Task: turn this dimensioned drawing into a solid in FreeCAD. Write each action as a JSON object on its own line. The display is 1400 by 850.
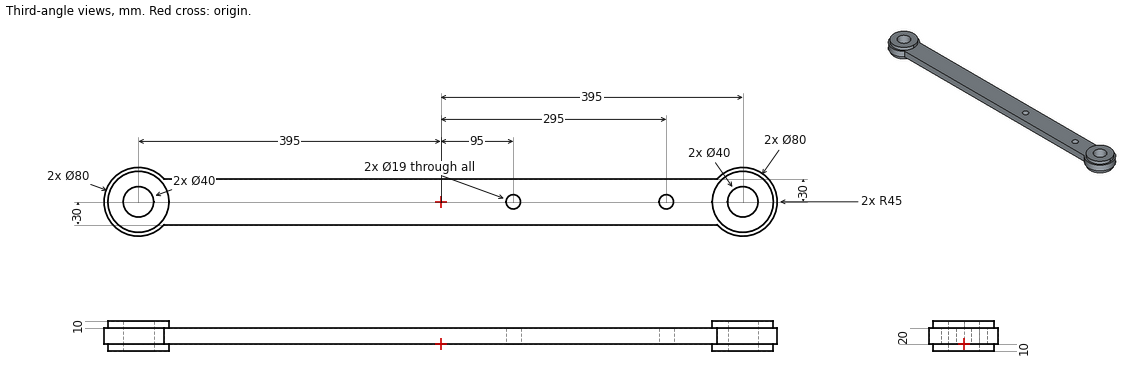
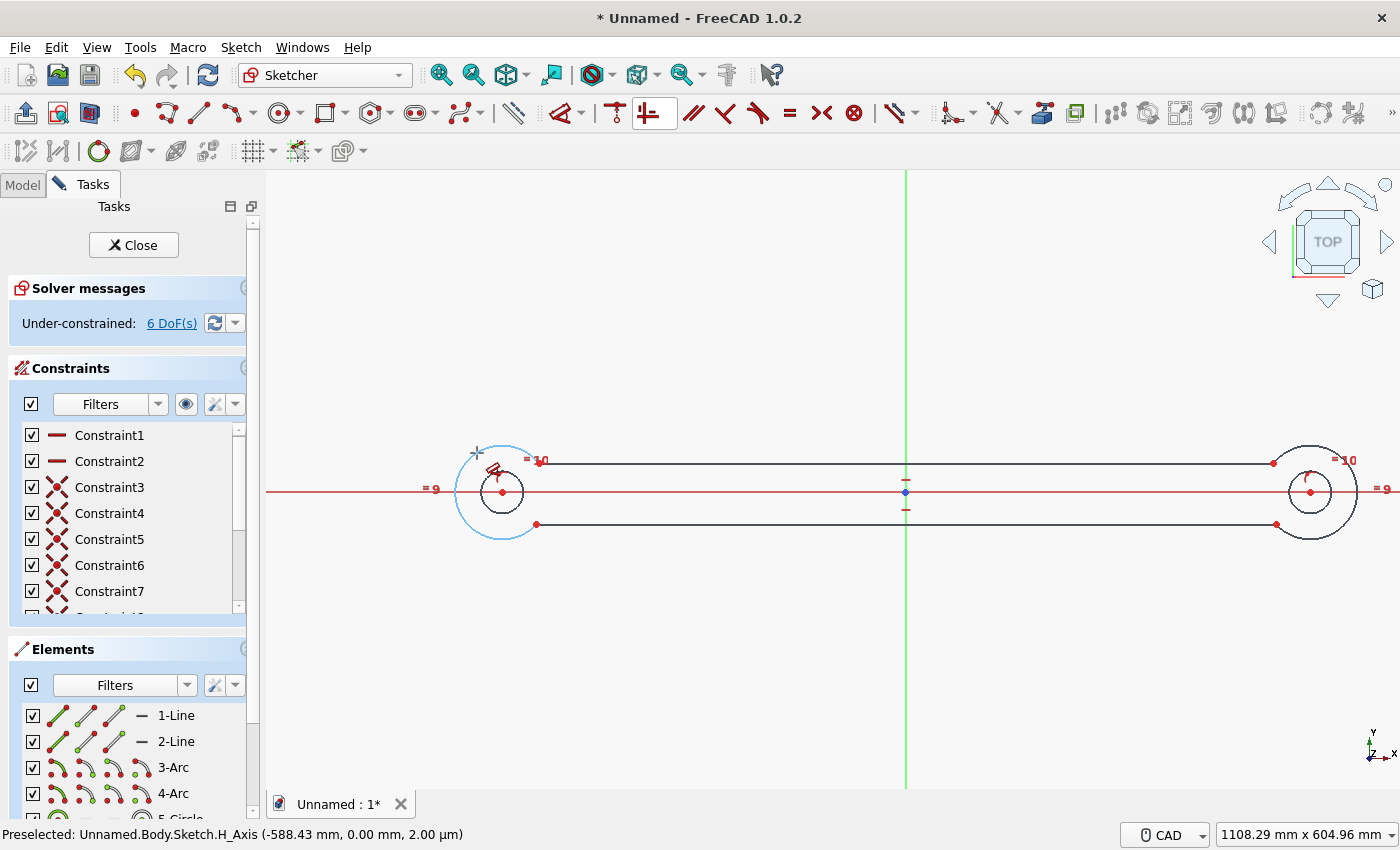
{"action": "left_click", "coordinate": [478, 453]}
{"action": "left_click", "coordinate": [461, 426]}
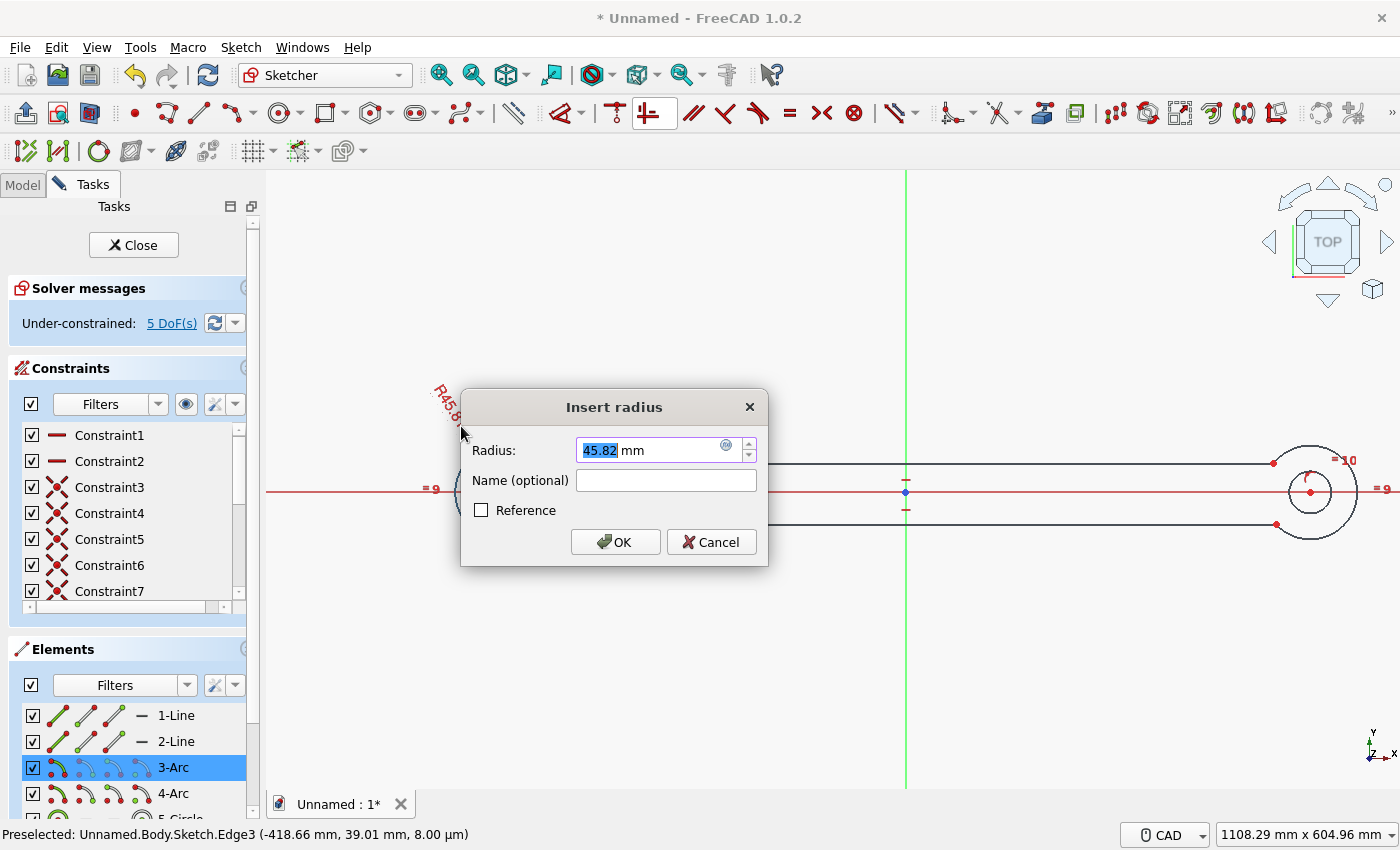
{"action": "type", "text": "45"}
{"action": "key", "text": "Return"}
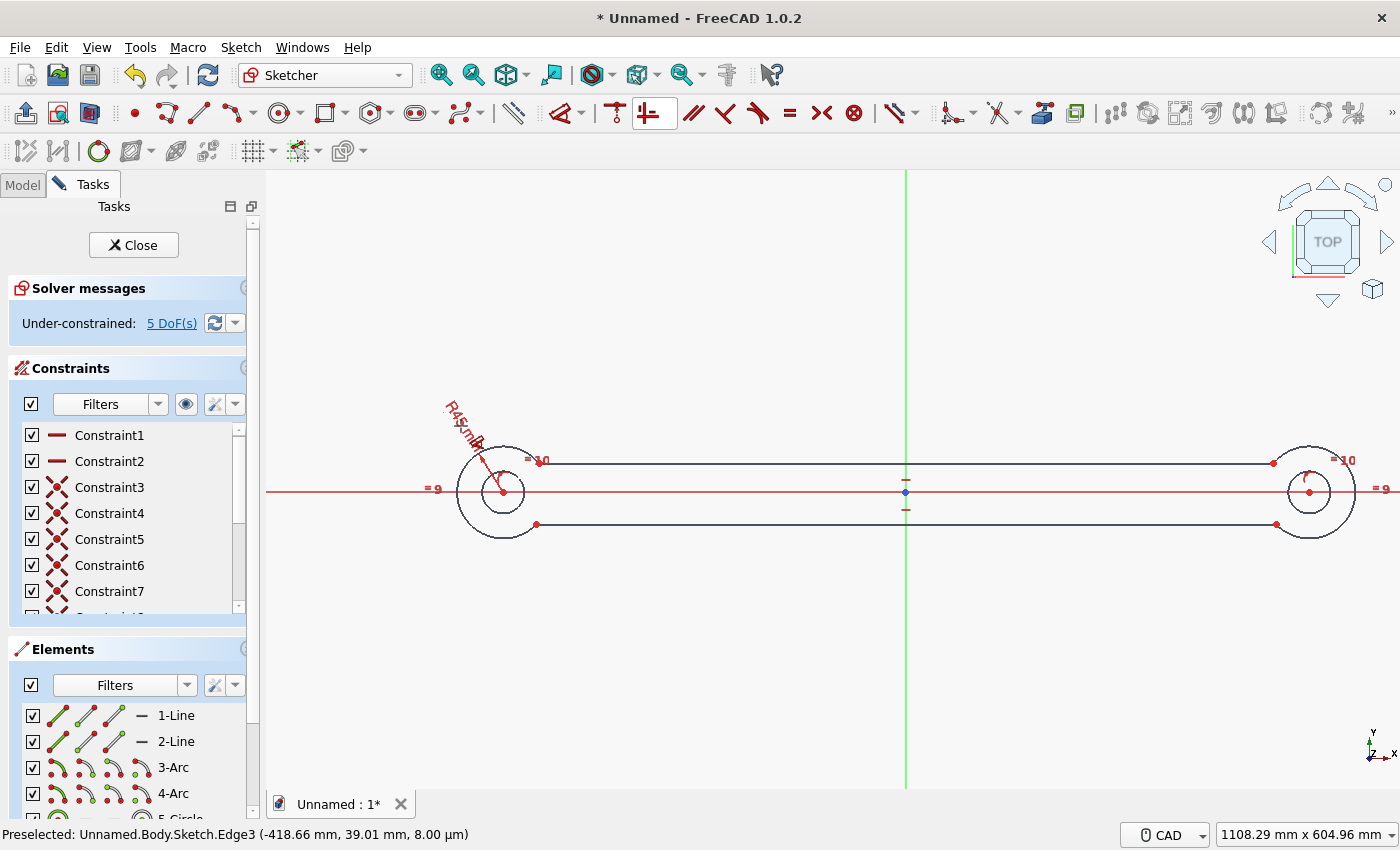
{"action": "left_click", "coordinate": [518, 478]}
{"action": "left_click", "coordinate": [554, 478]}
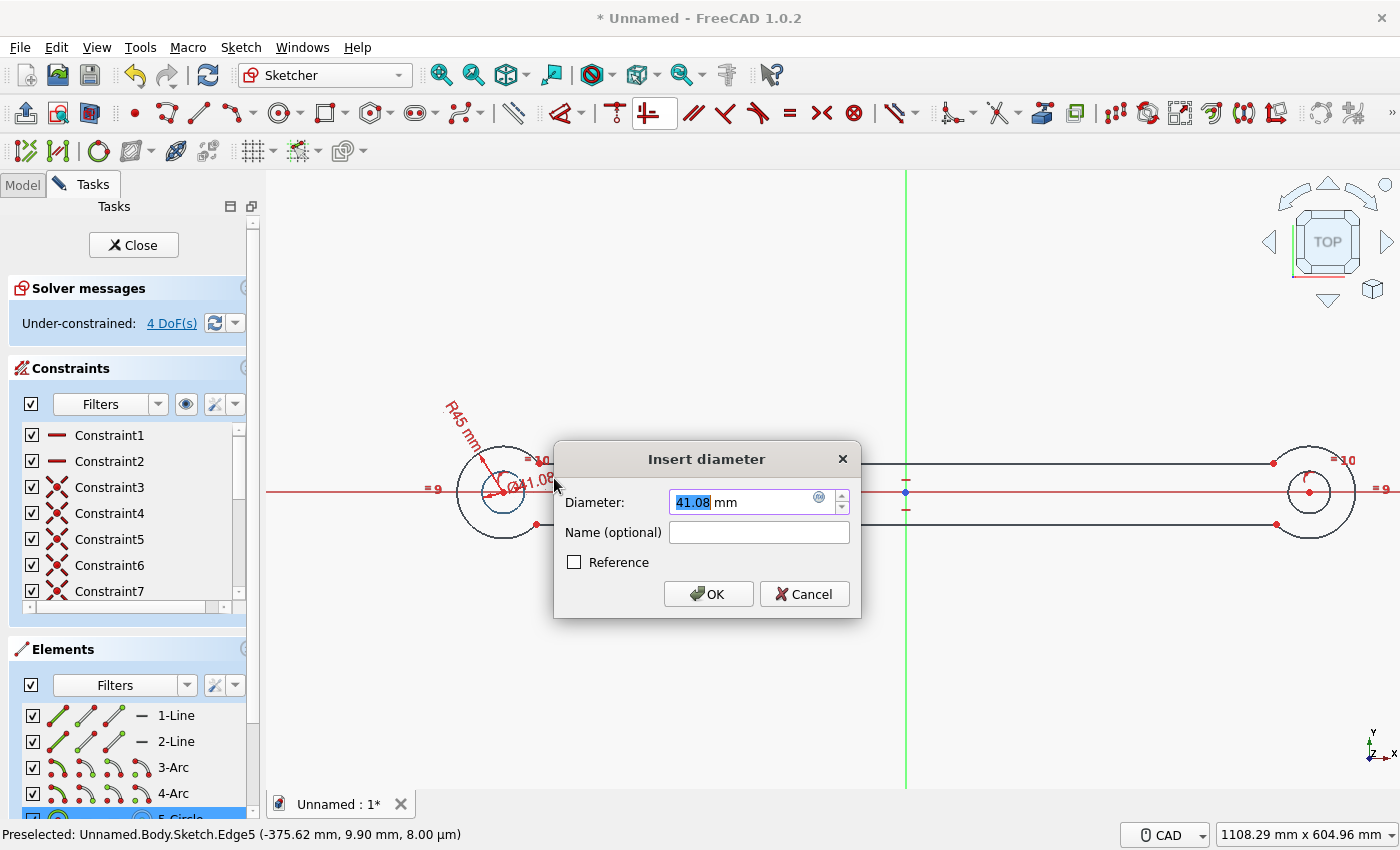
{"action": "type", "text": "40"}
{"action": "key", "text": "Return"}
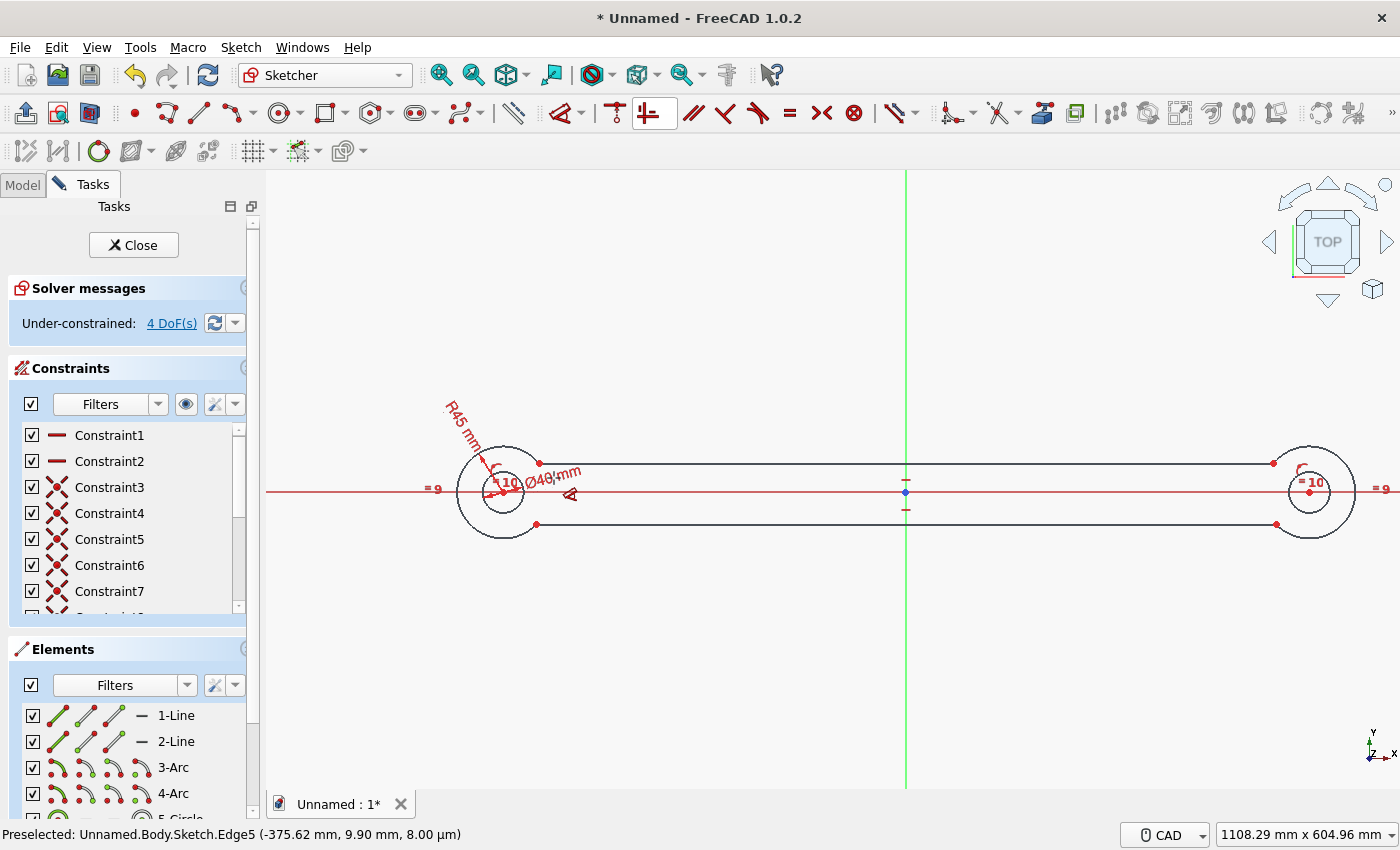
{"action": "scroll", "coordinate": [477, 453], "scroll_direction": "down", "scroll_amount": 2}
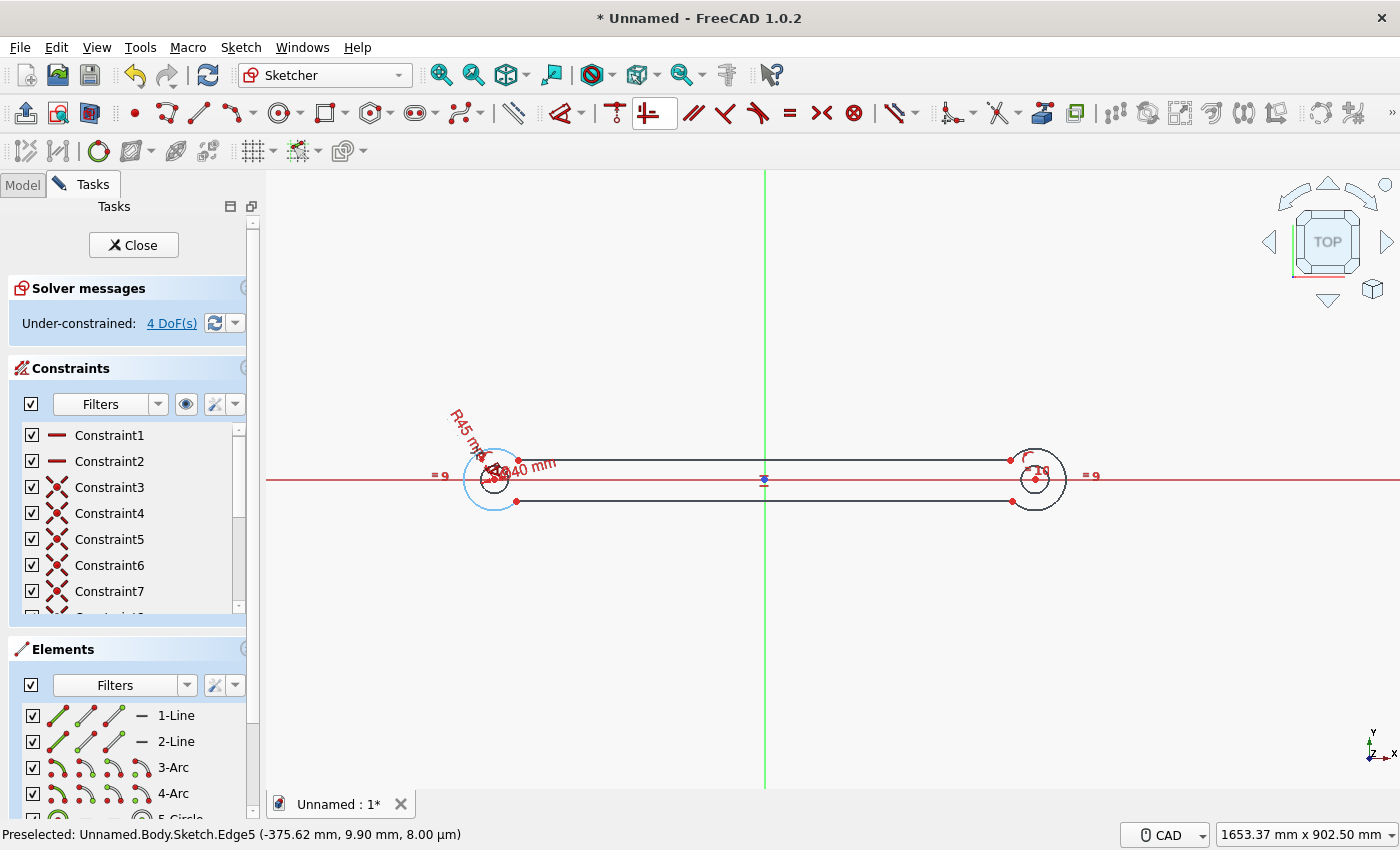
{"action": "scroll", "coordinate": [1011, 460], "scroll_direction": "up", "scroll_amount": 4}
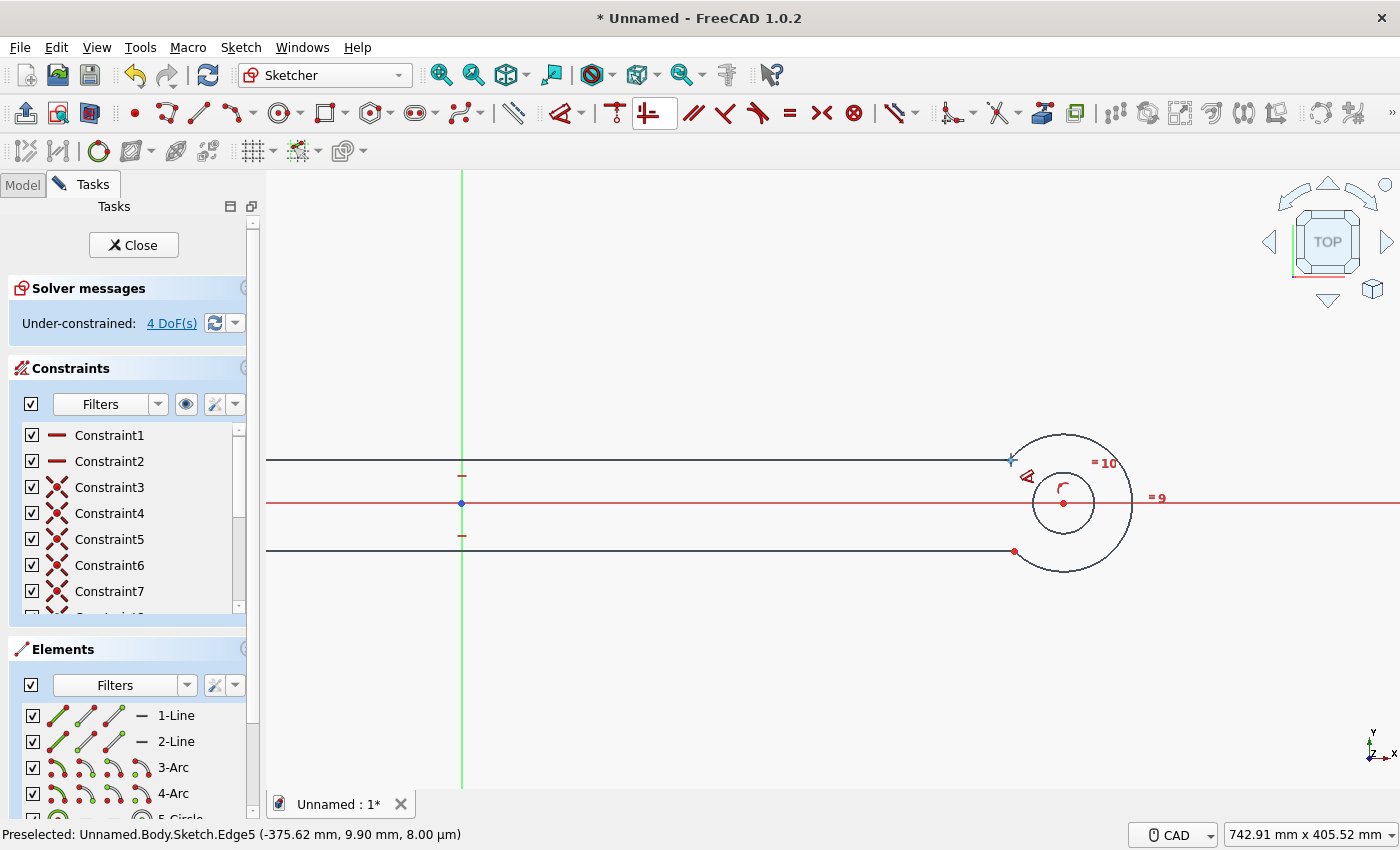
{"action": "left_click", "coordinate": [1010, 460]}
{"action": "left_click", "coordinate": [428, 482]}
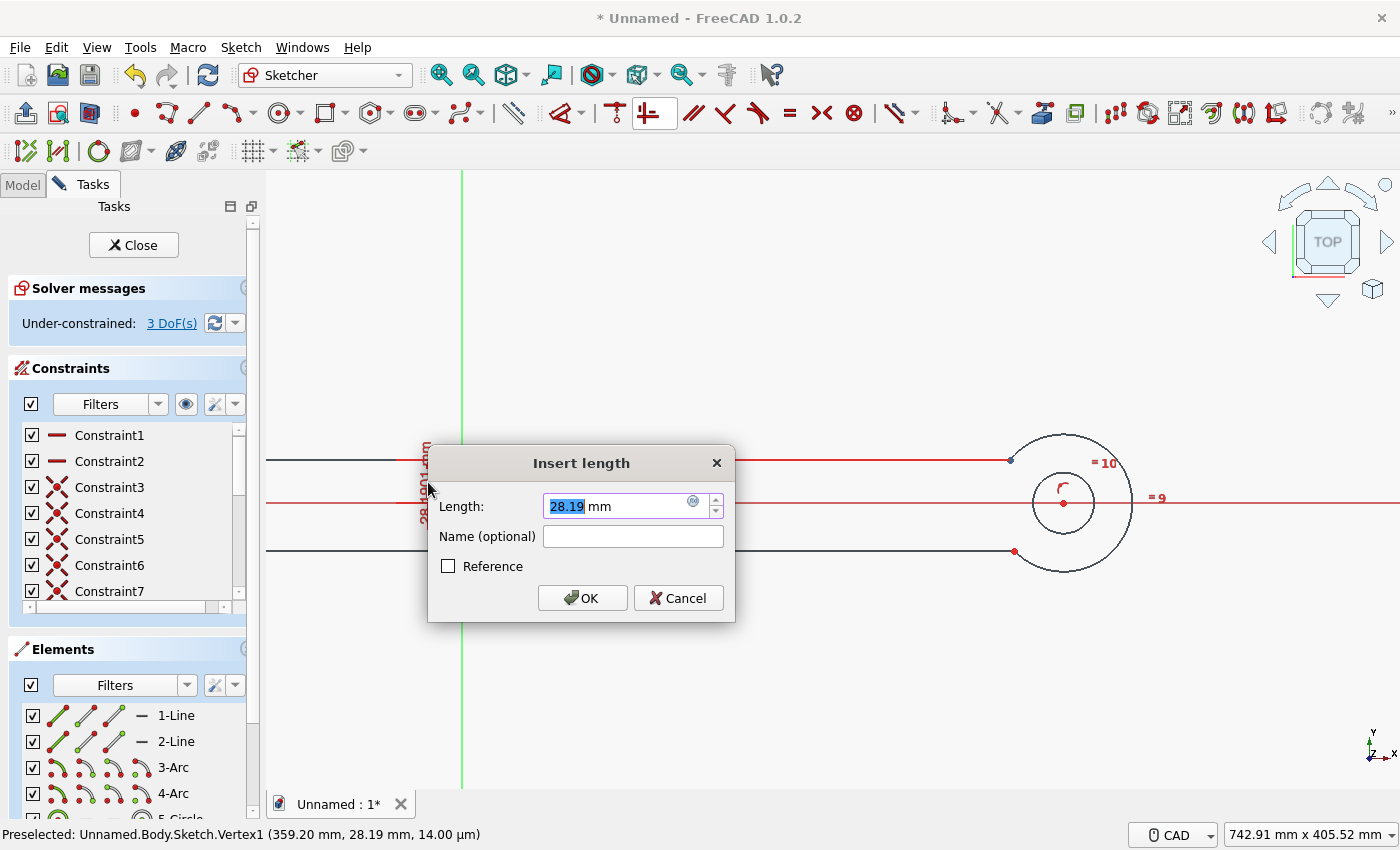
{"action": "type", "text": "30"}
{"action": "key", "text": "Return"}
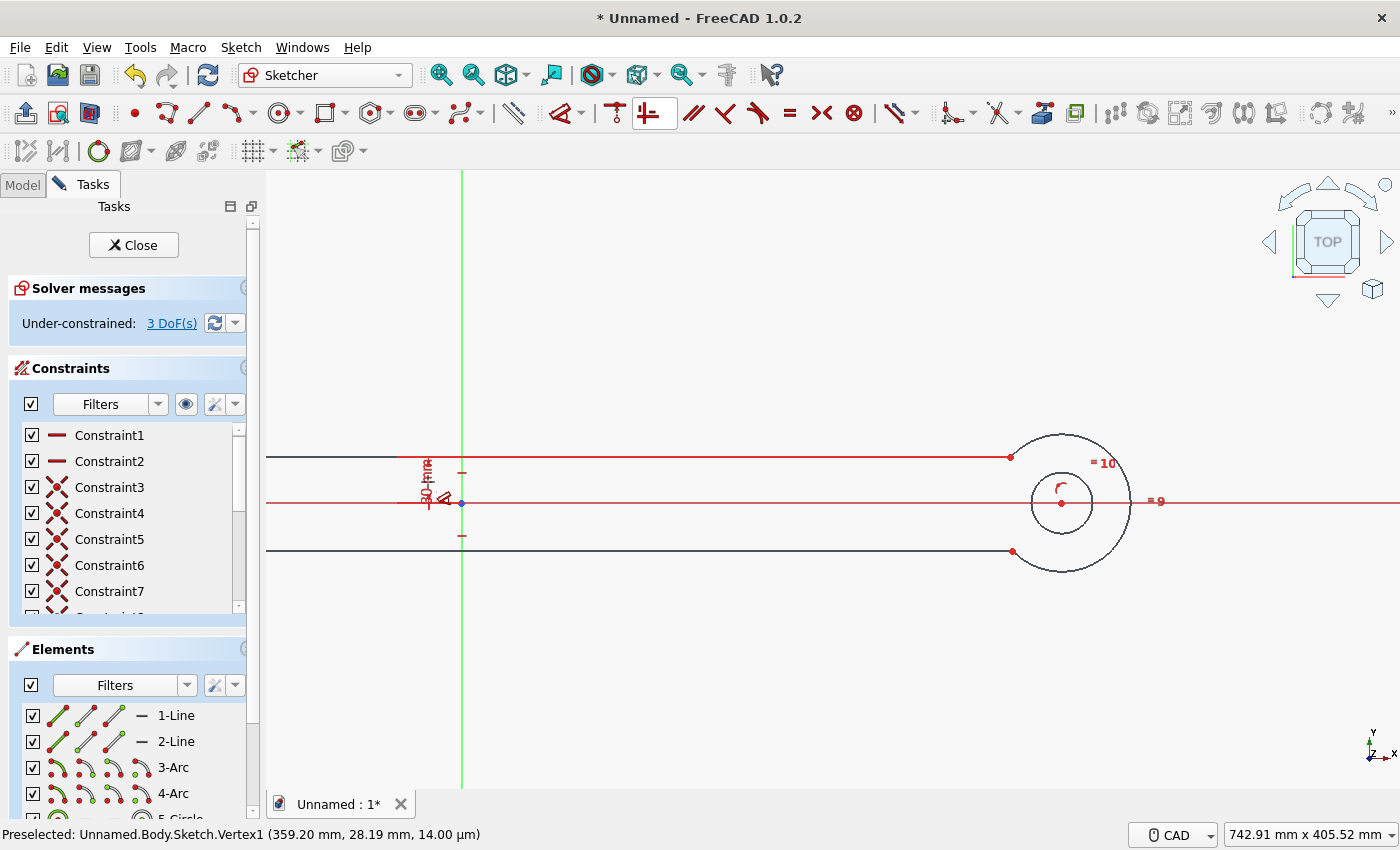
{"action": "scroll", "coordinate": [1012, 460], "scroll_direction": "down", "scroll_amount": 4}